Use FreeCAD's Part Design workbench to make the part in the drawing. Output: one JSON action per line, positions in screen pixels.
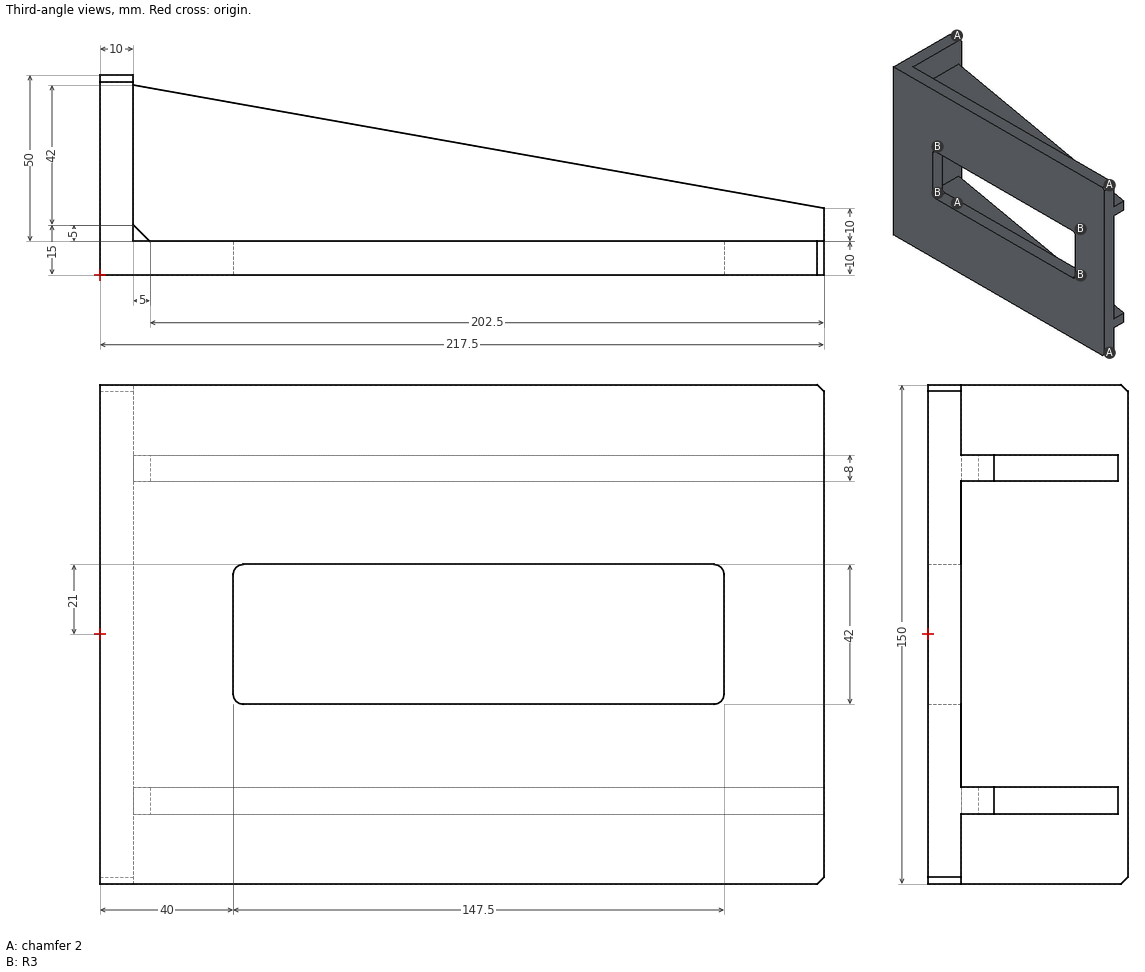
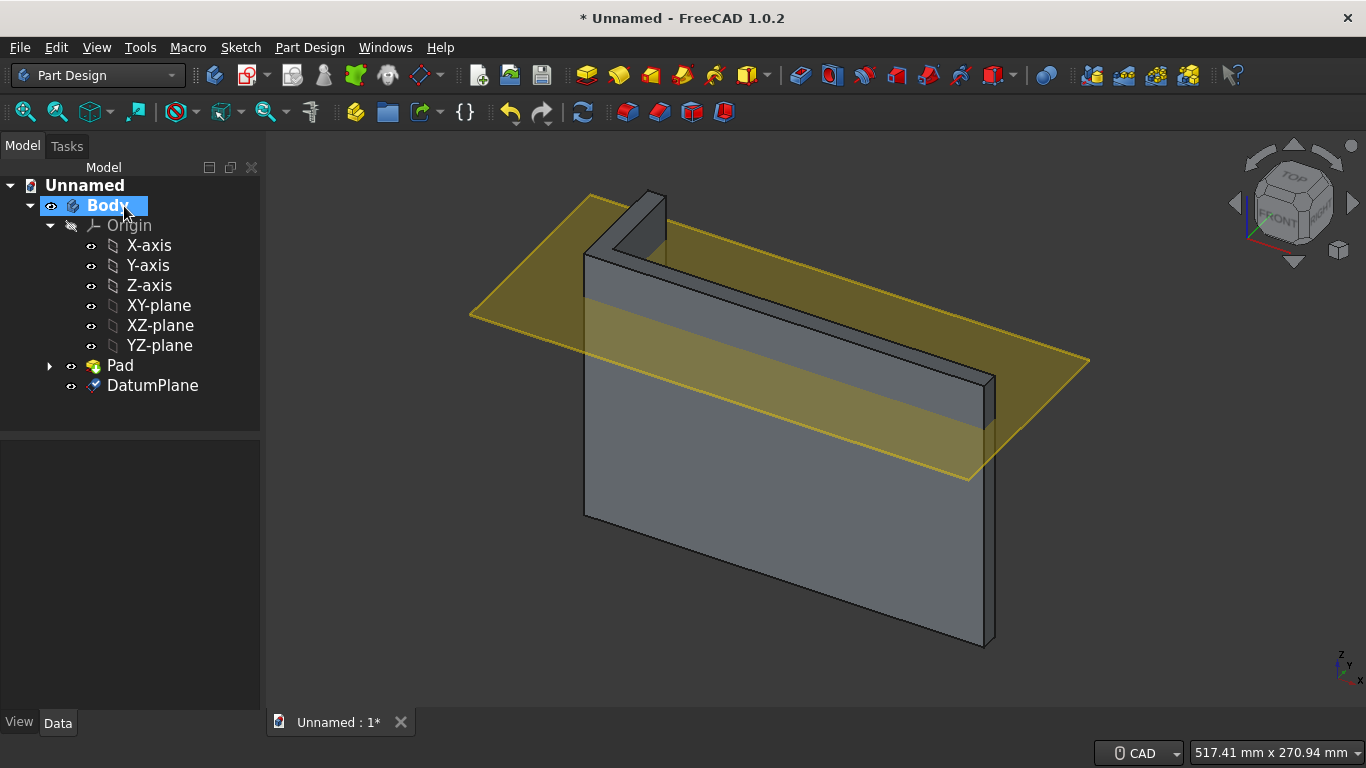
{"action": "left_click", "coordinate": [116, 386]}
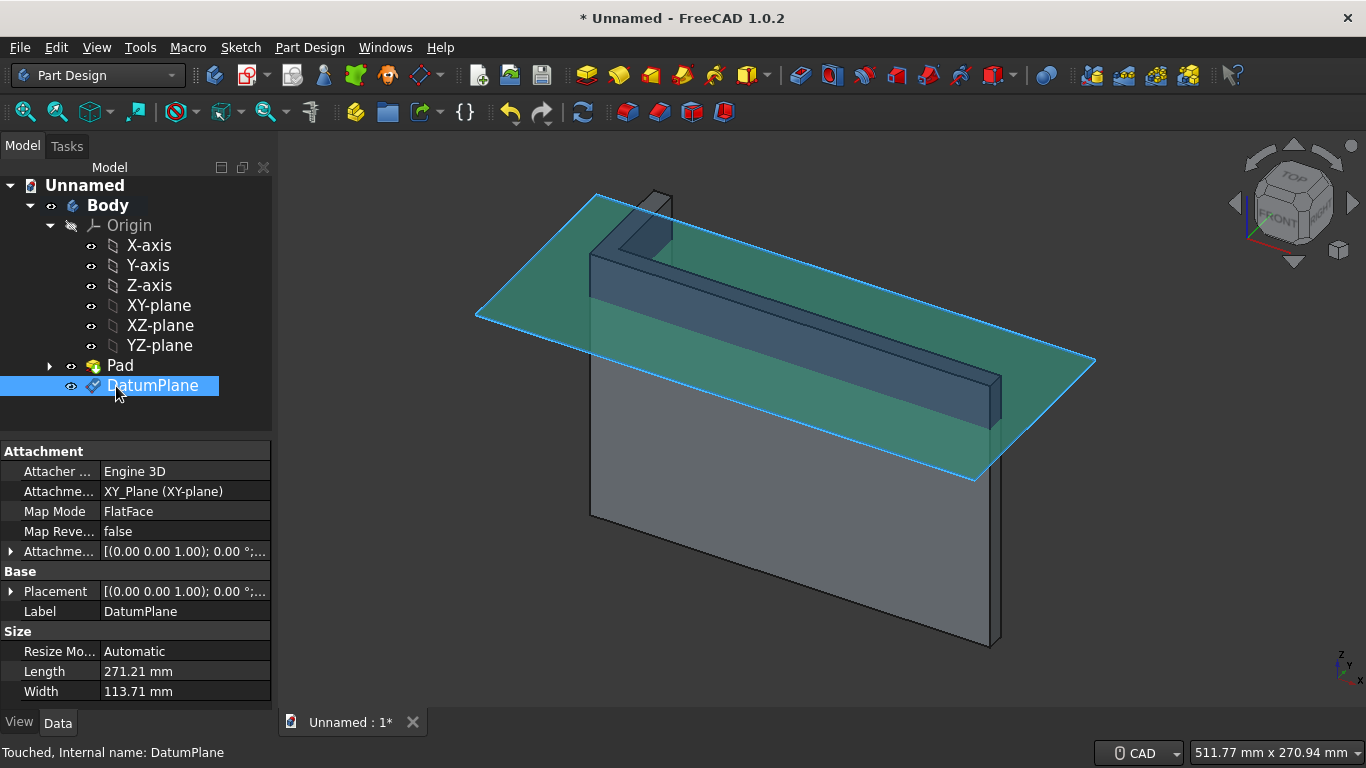
{"action": "left_click", "coordinate": [248, 76]}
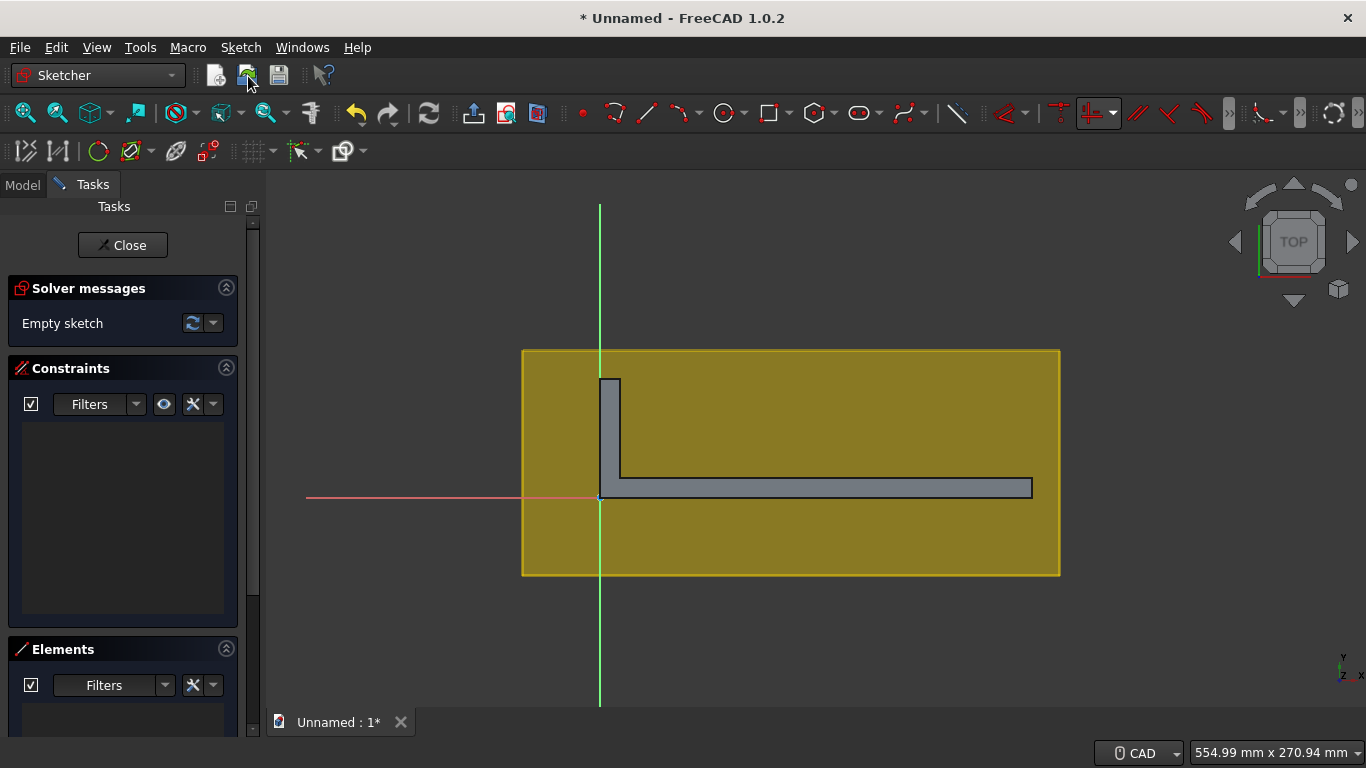
{"action": "left_click", "coordinate": [538, 114]}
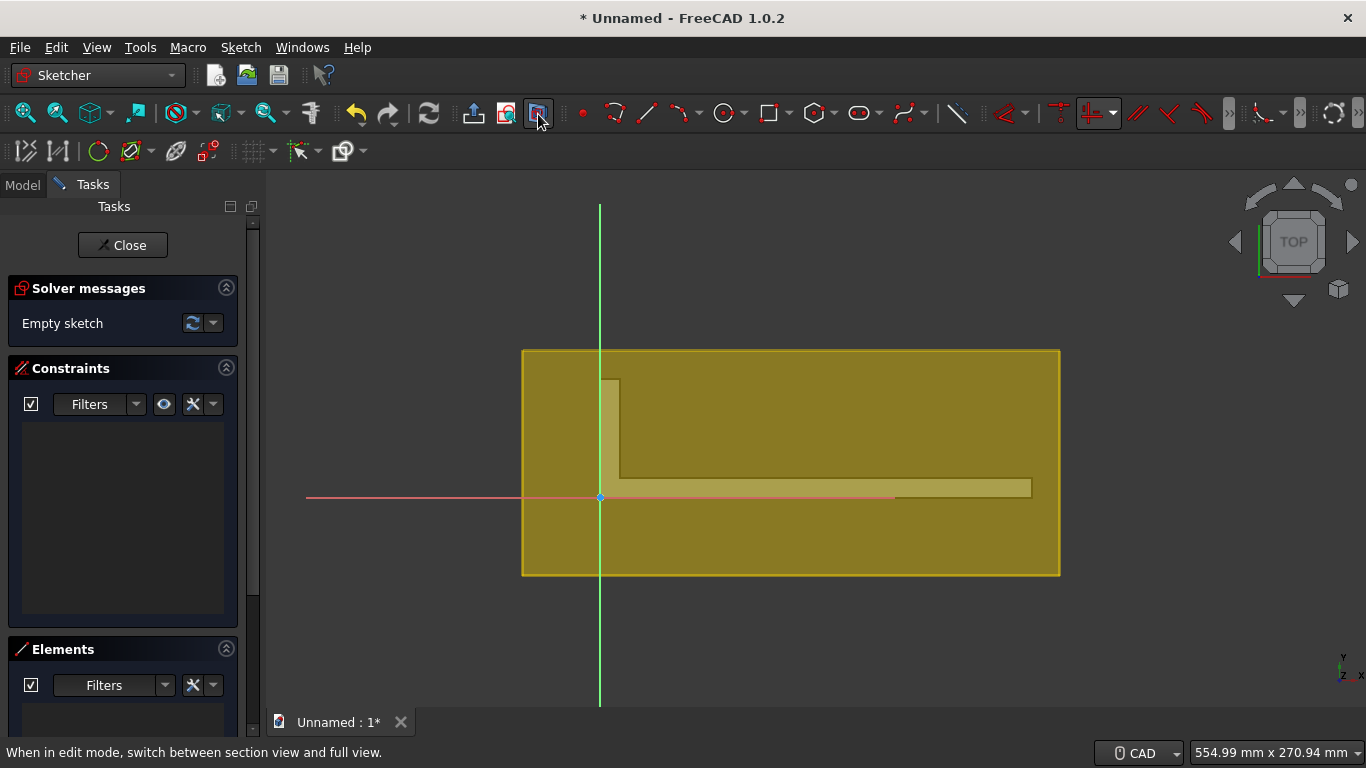
{"action": "scroll", "coordinate": [955, 448], "scroll_direction": "up", "scroll_amount": 2}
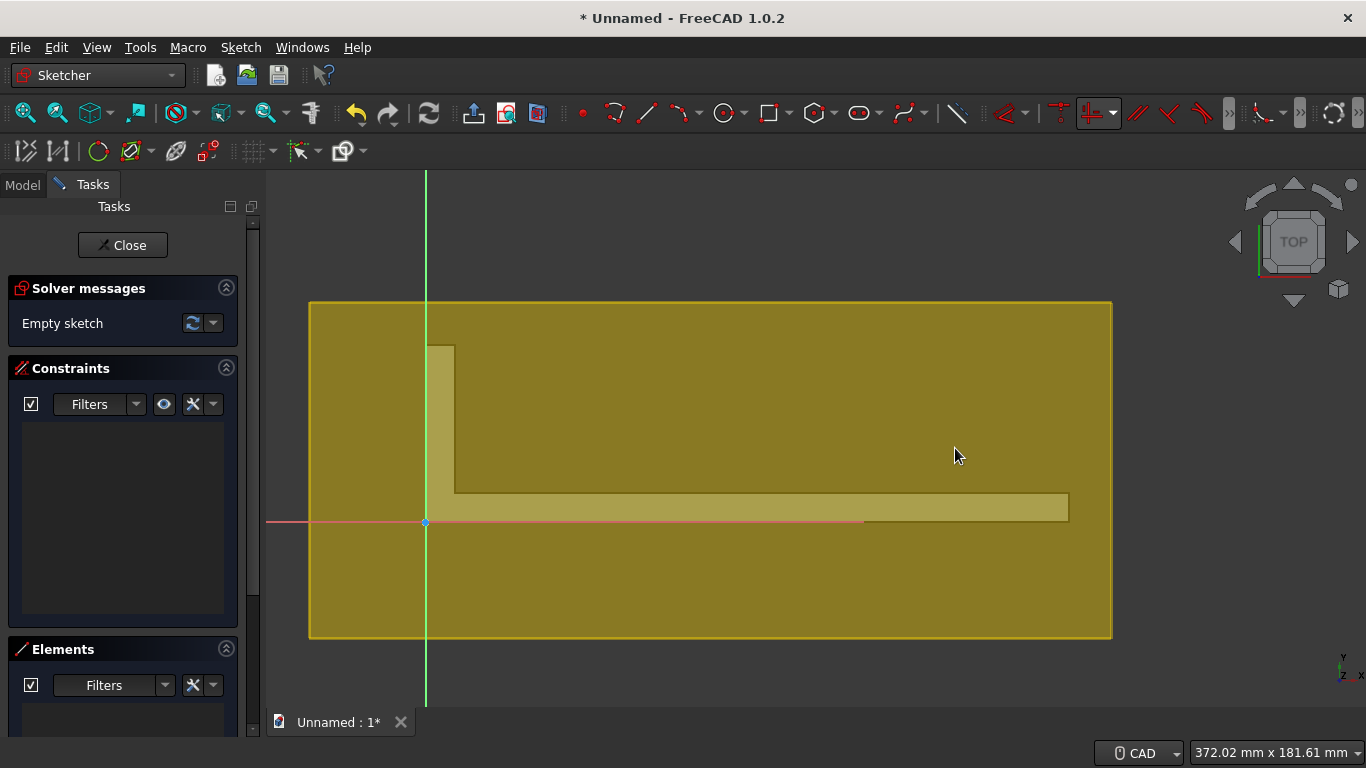
{"action": "left_click", "coordinate": [616, 114]}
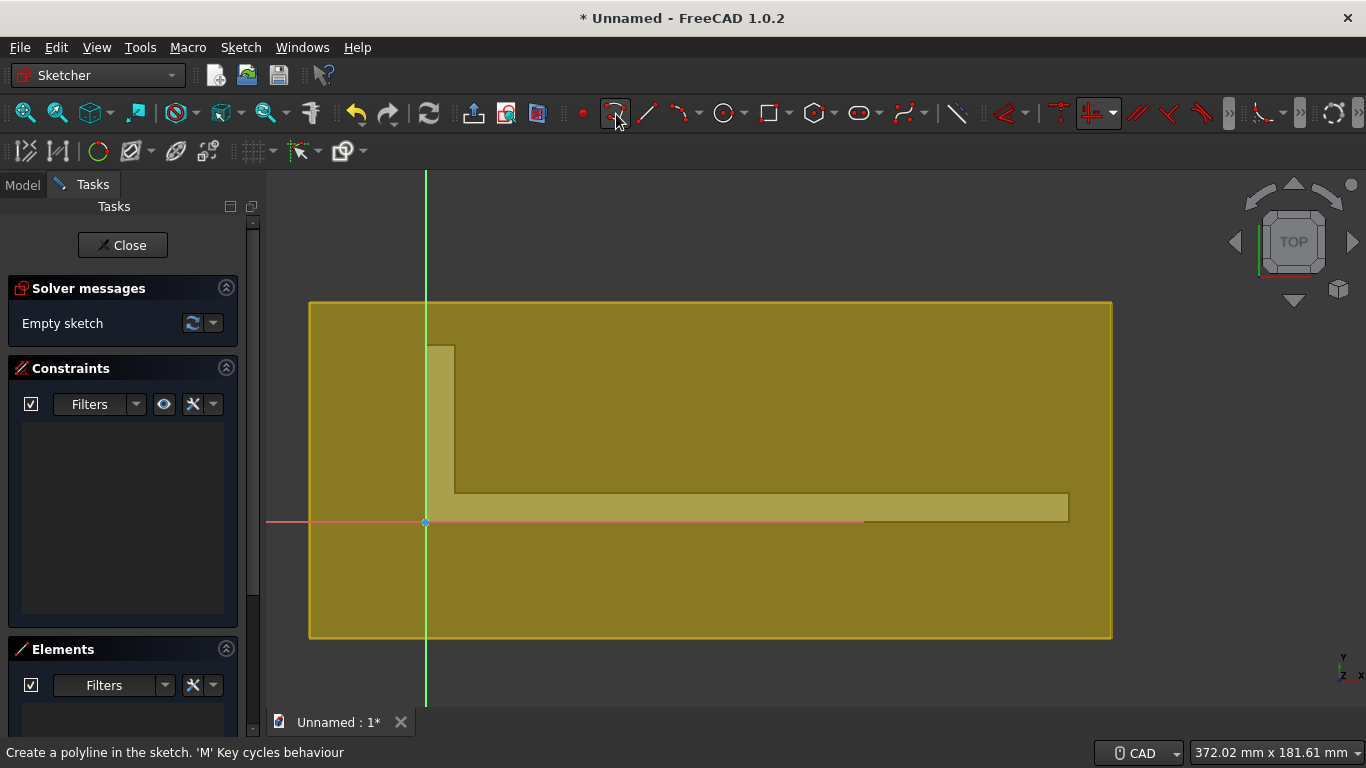
{"action": "left_click", "coordinate": [455, 478]}
{"action": "left_click", "coordinate": [470, 493]}
{"action": "left_click", "coordinate": [1069, 493]}
{"action": "left_click", "coordinate": [1069, 463]}
{"action": "left_click", "coordinate": [455, 354]}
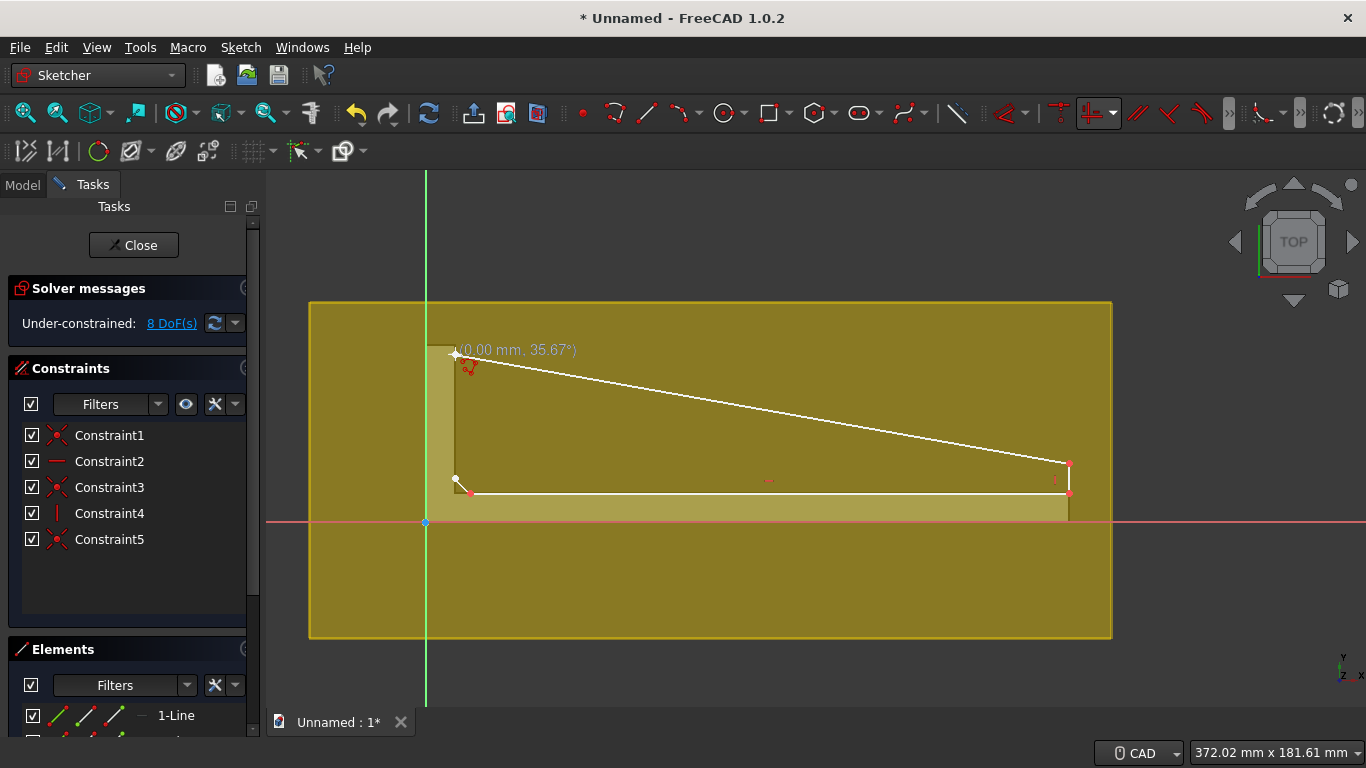
{"action": "scroll", "coordinate": [455, 478], "scroll_direction": "up", "scroll_amount": 3}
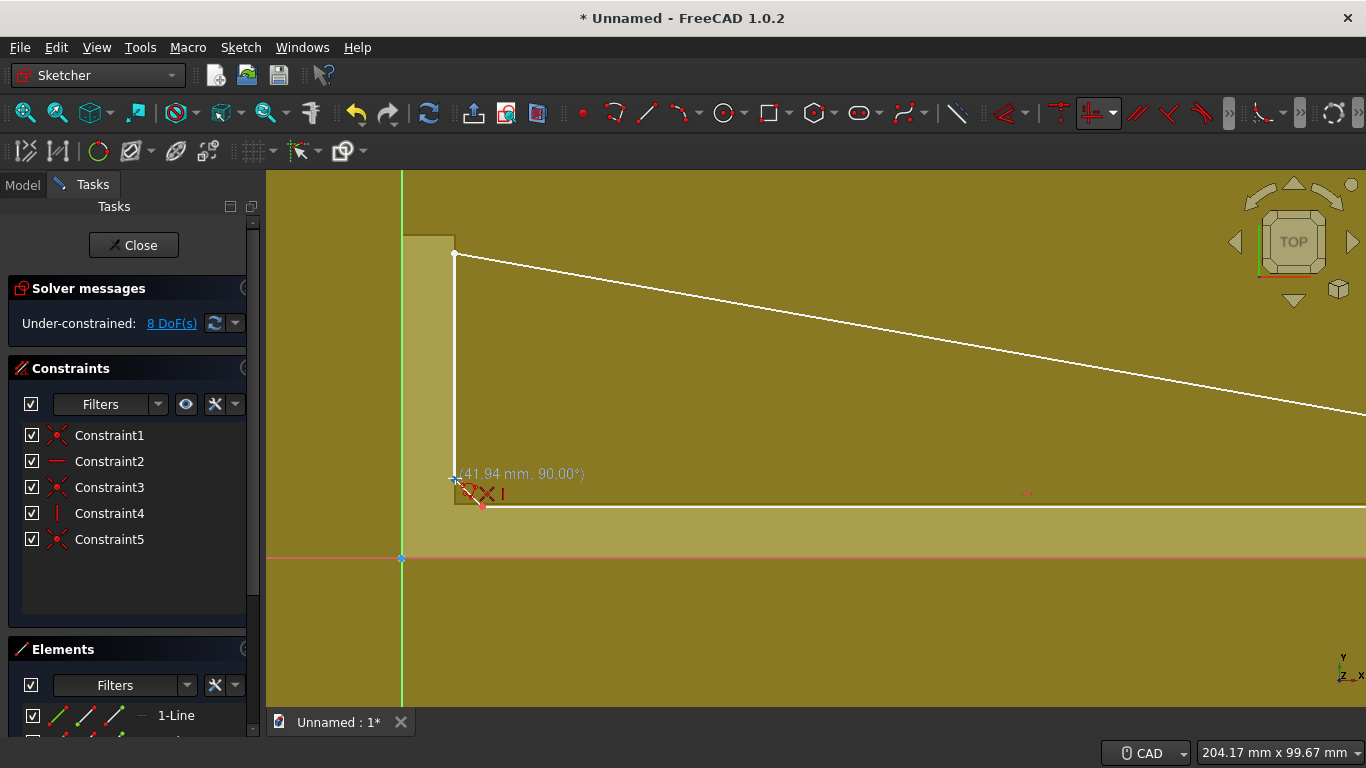
{"action": "left_click", "coordinate": [455, 479]}
{"action": "key", "text": "Escape"}
{"action": "key", "text": "Escape"}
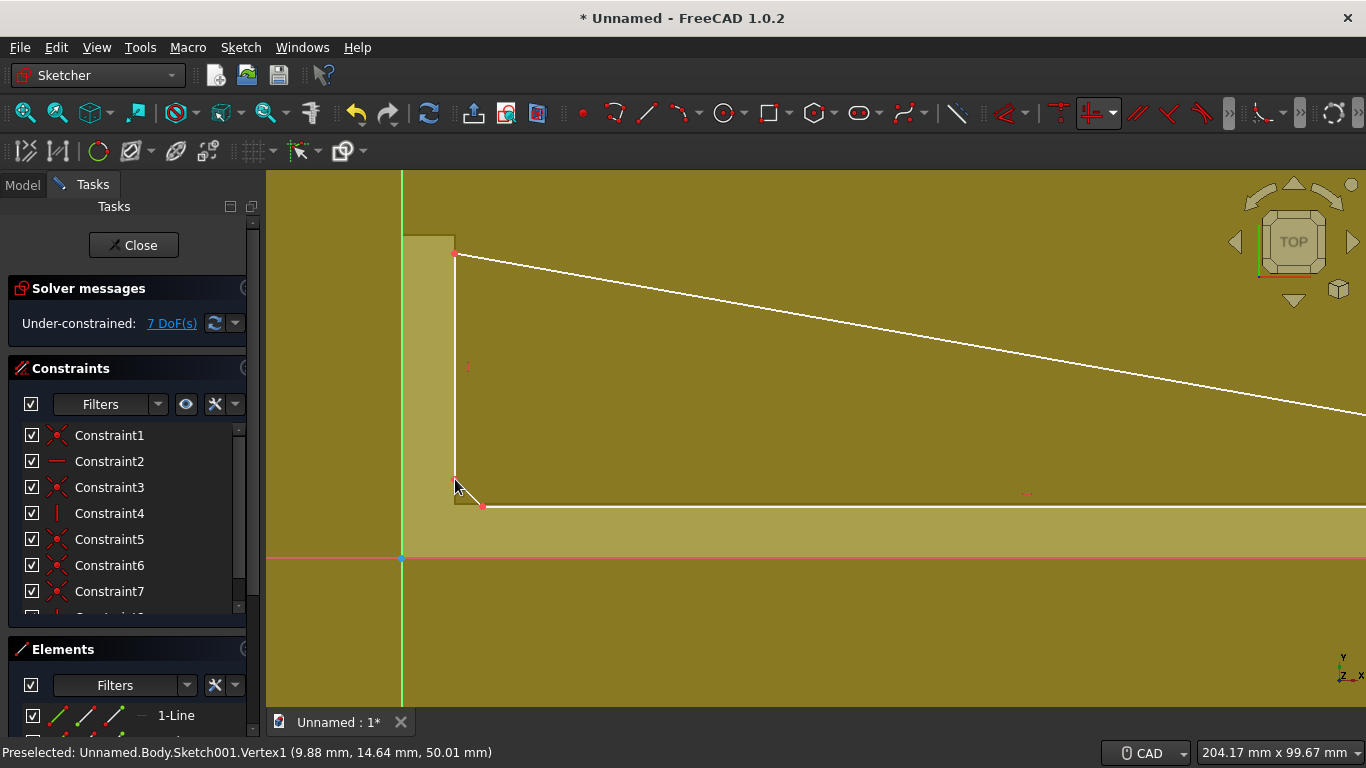
{"action": "left_click", "coordinate": [1004, 114]}